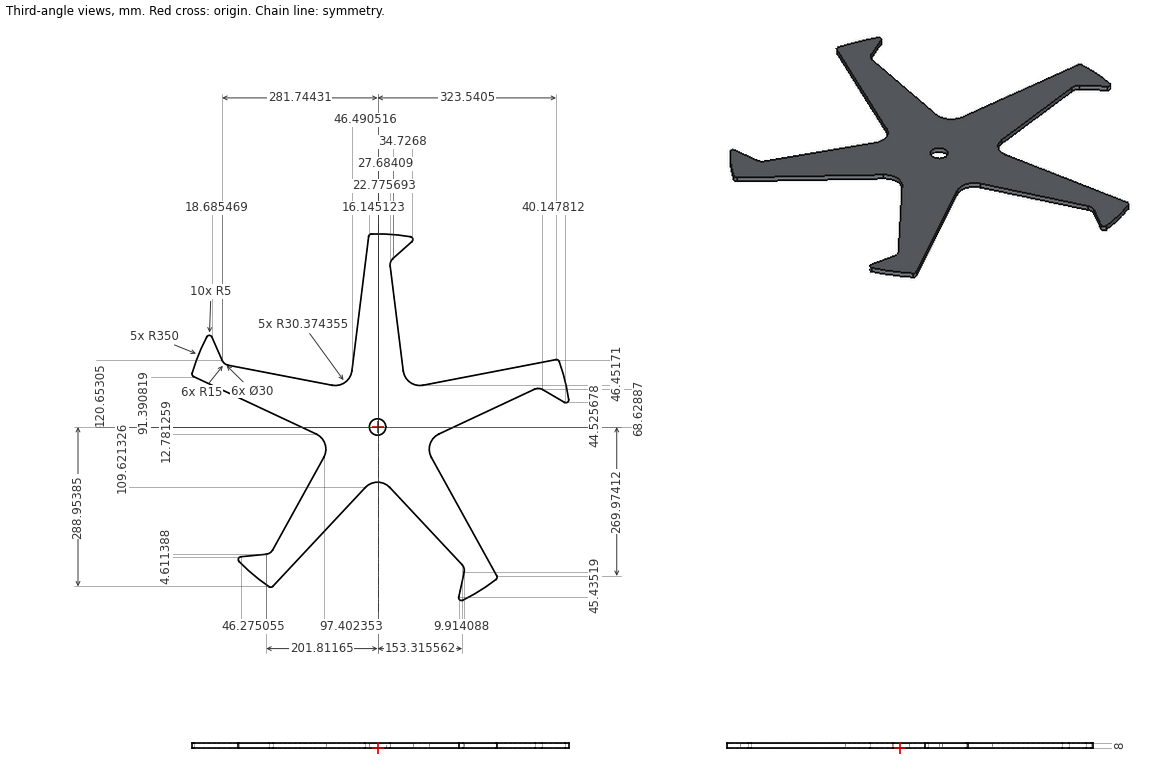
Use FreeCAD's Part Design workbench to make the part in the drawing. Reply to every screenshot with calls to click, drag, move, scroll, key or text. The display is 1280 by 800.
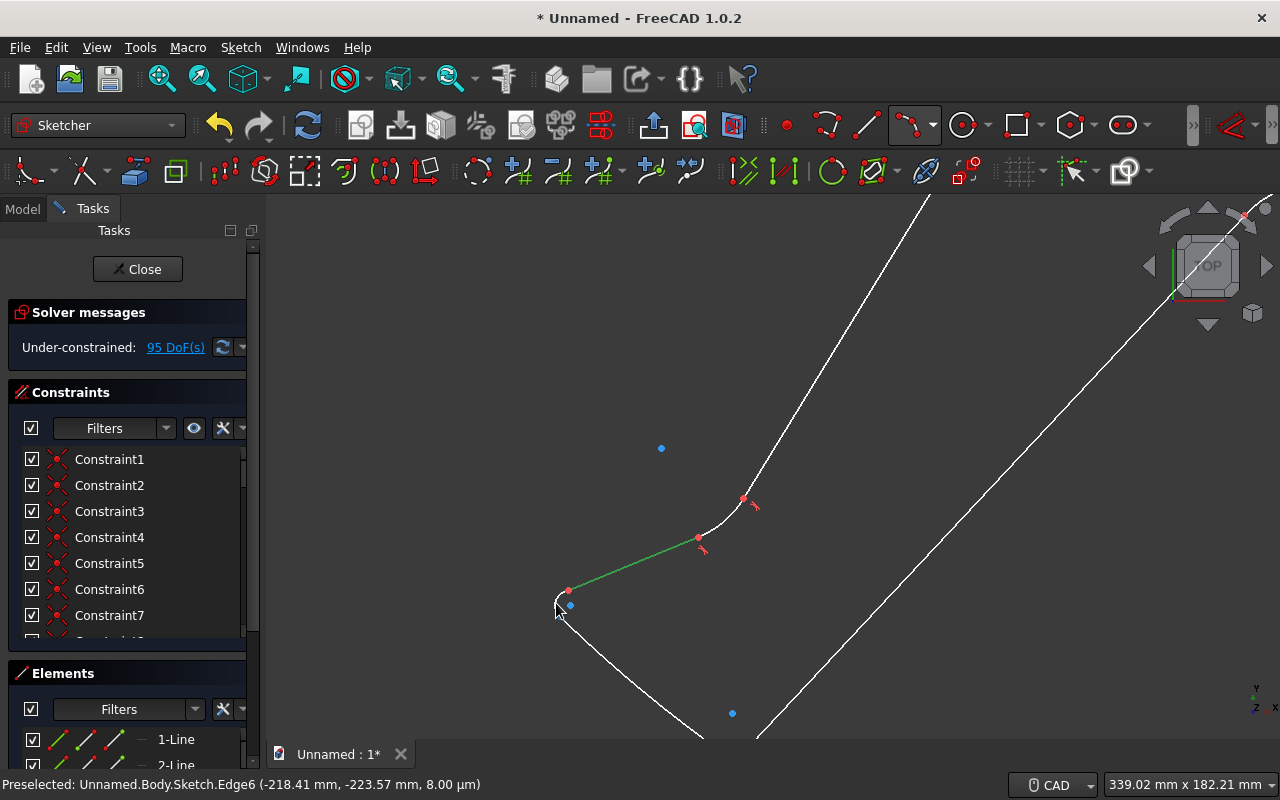
click(556, 601)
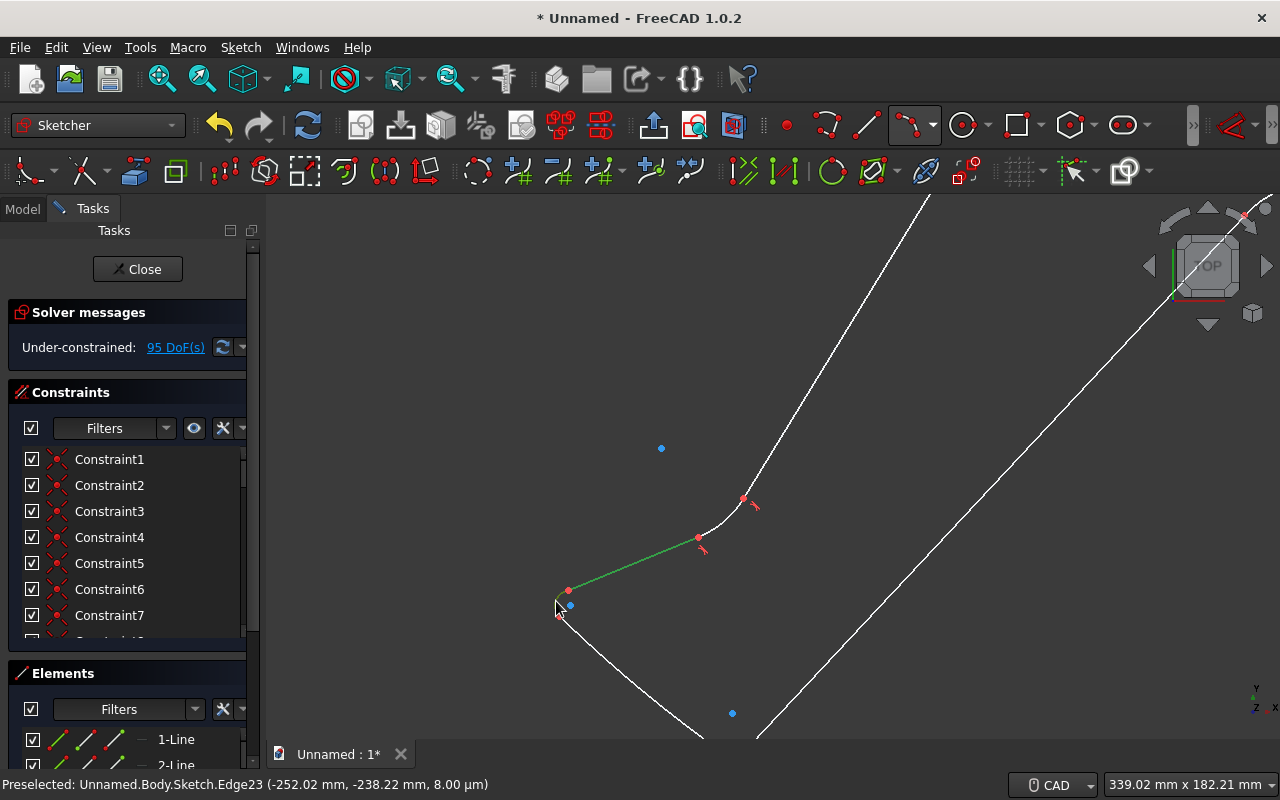
key(t)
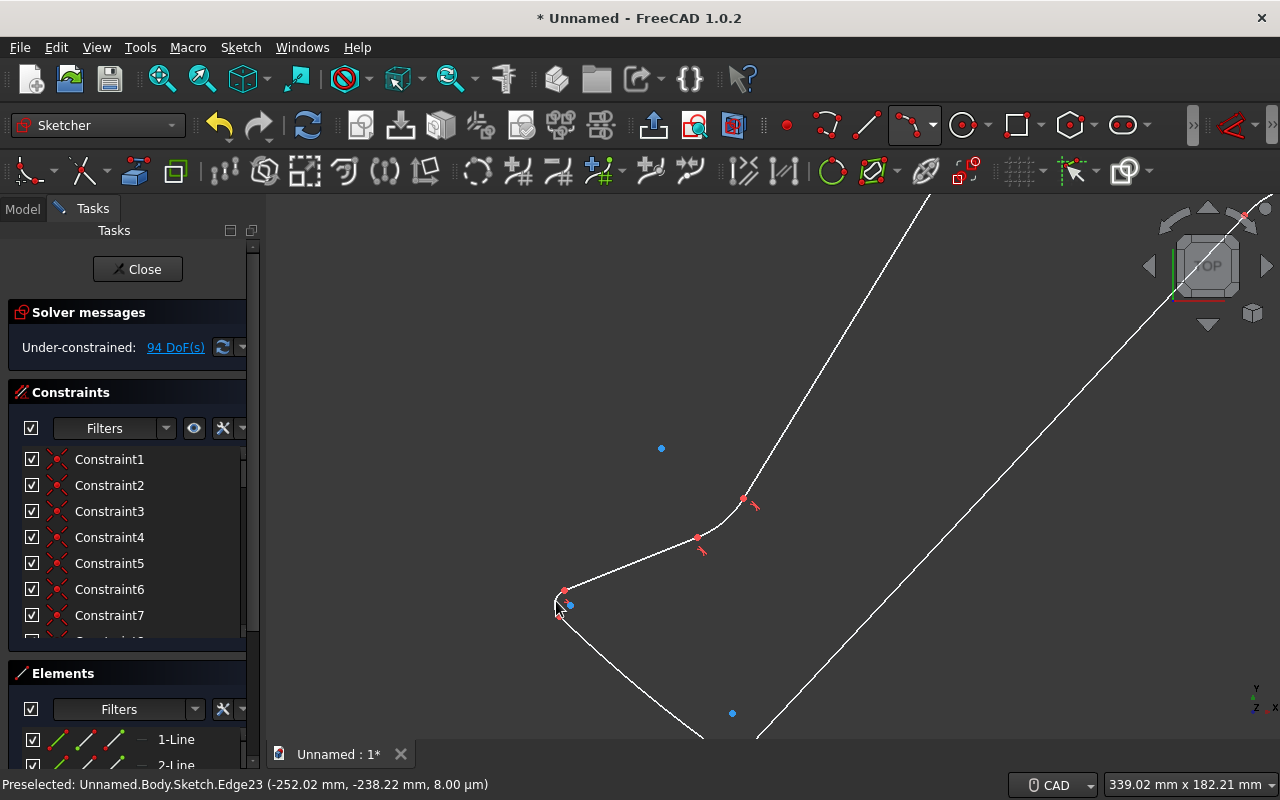
scroll(581, 592, down, 9)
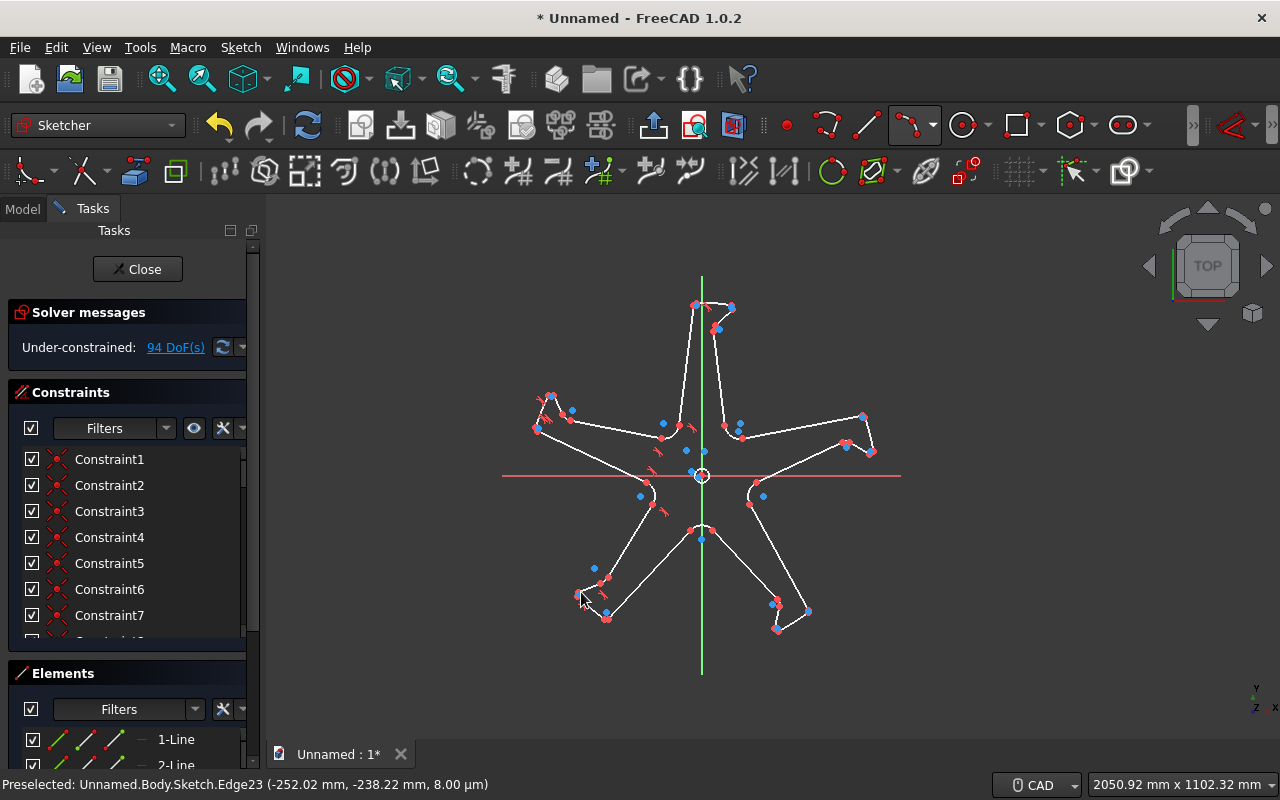
click(633, 593)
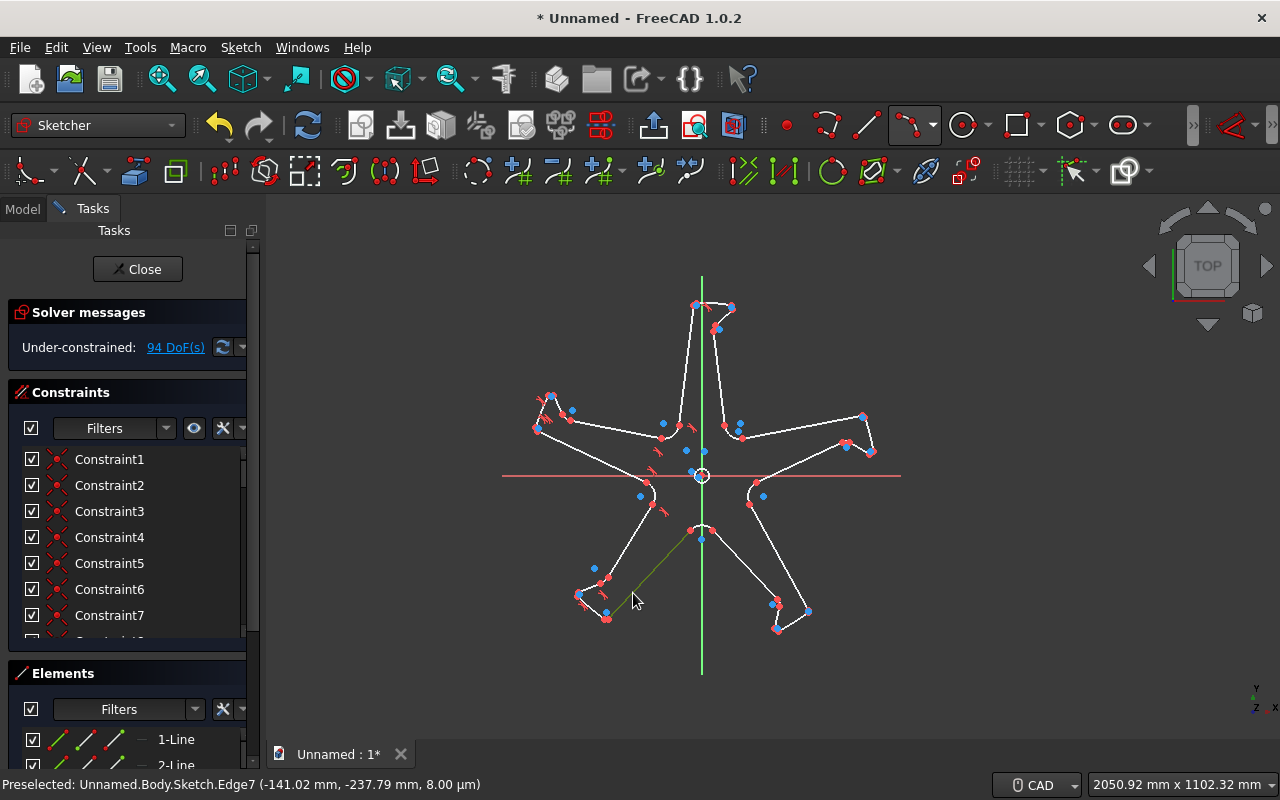
scroll(606, 619, up, 11)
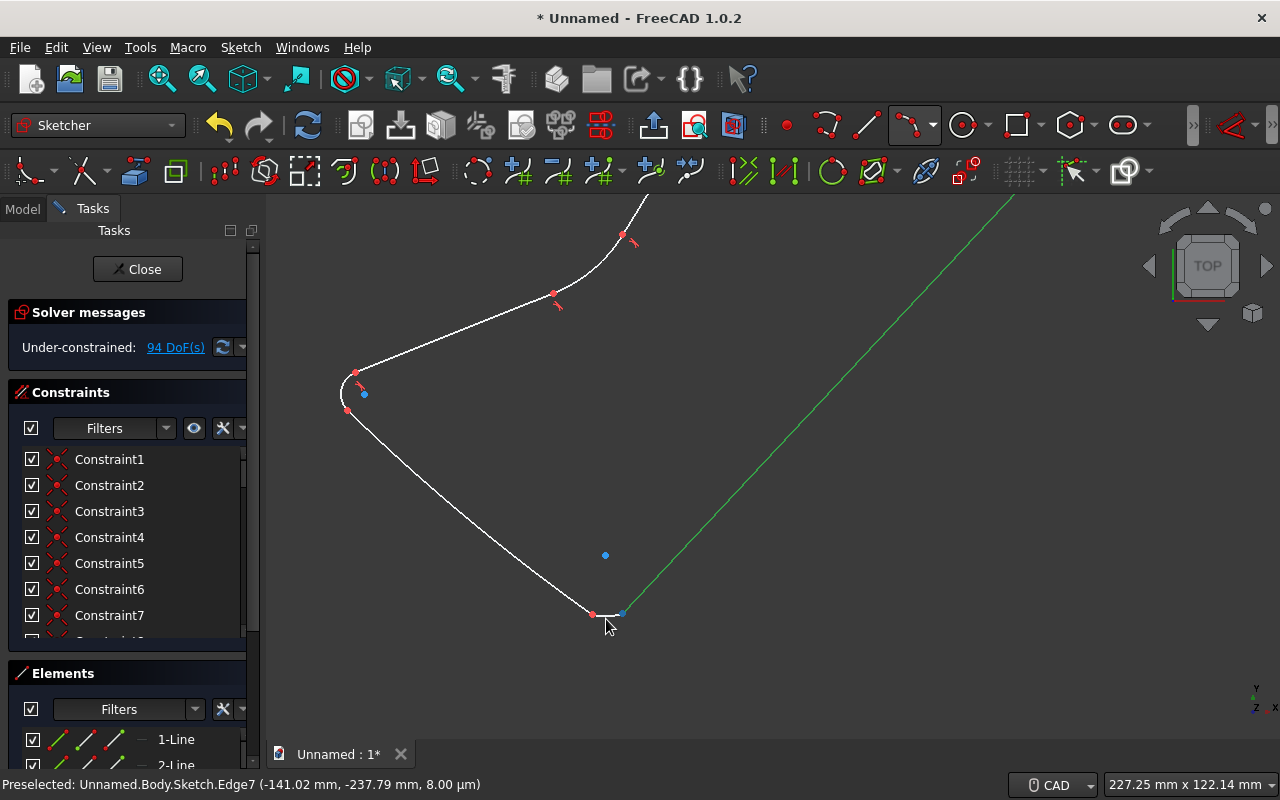
click(607, 616)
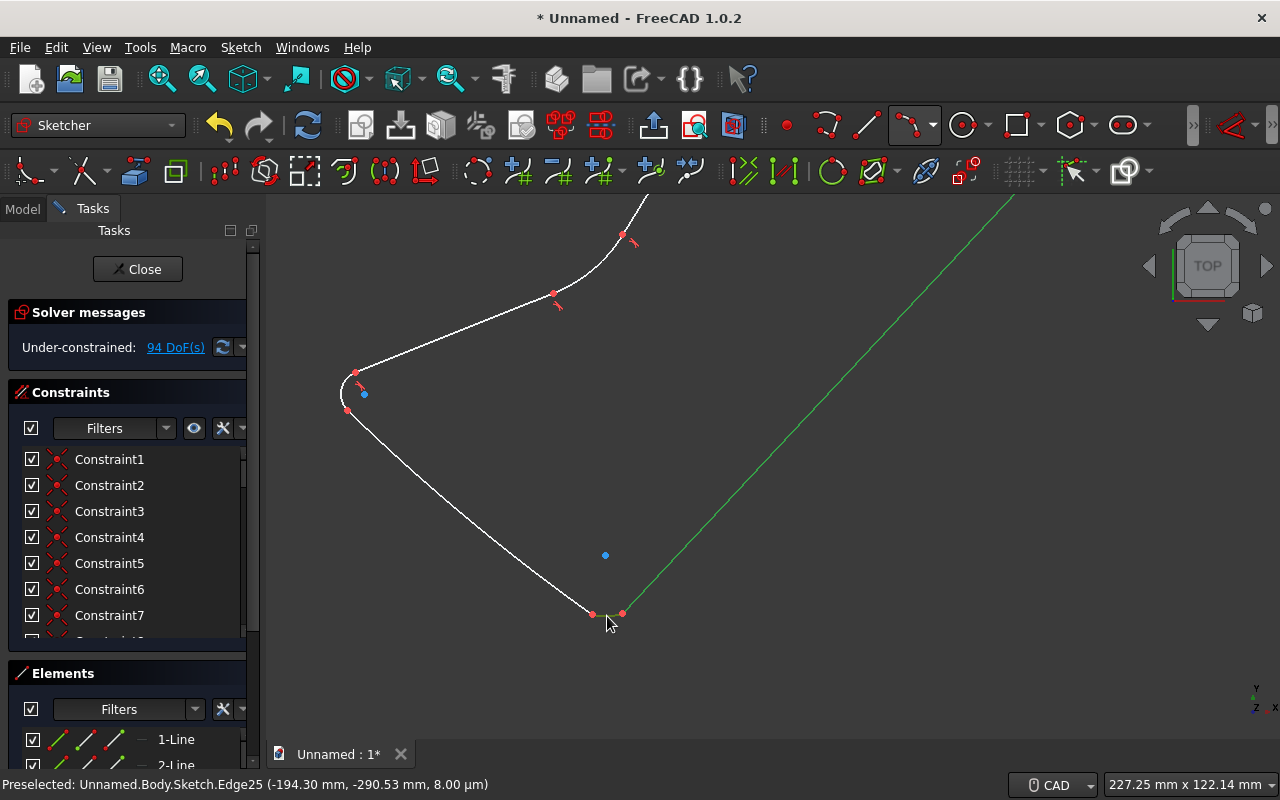
key(t)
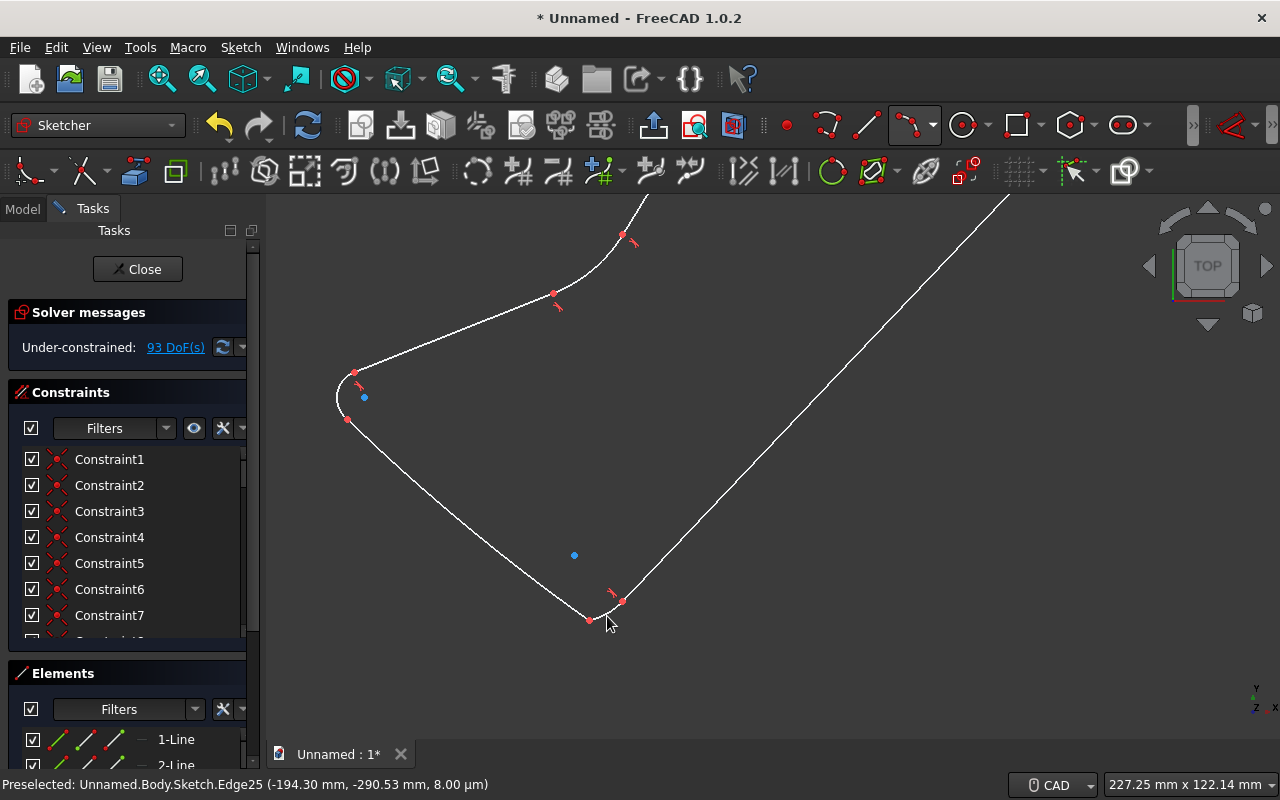
scroll(606, 619, down, 11)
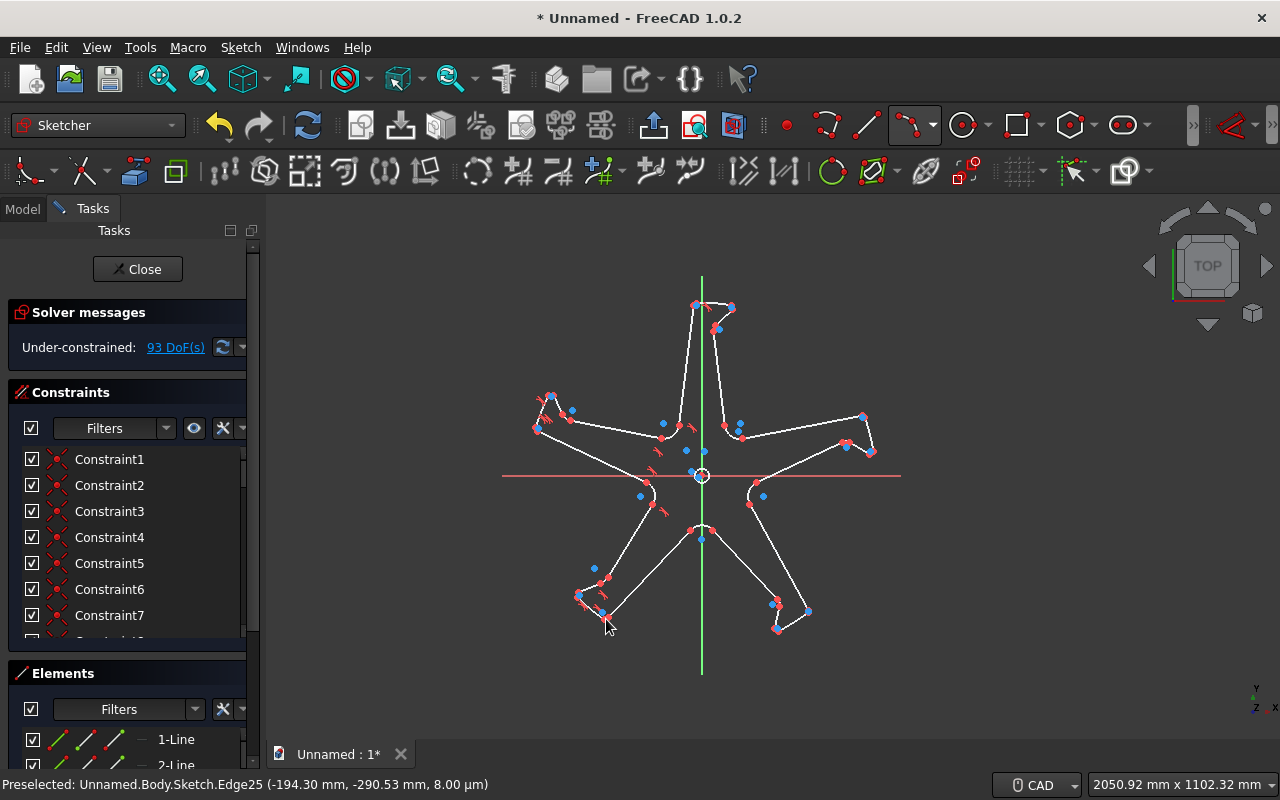
click(633, 592)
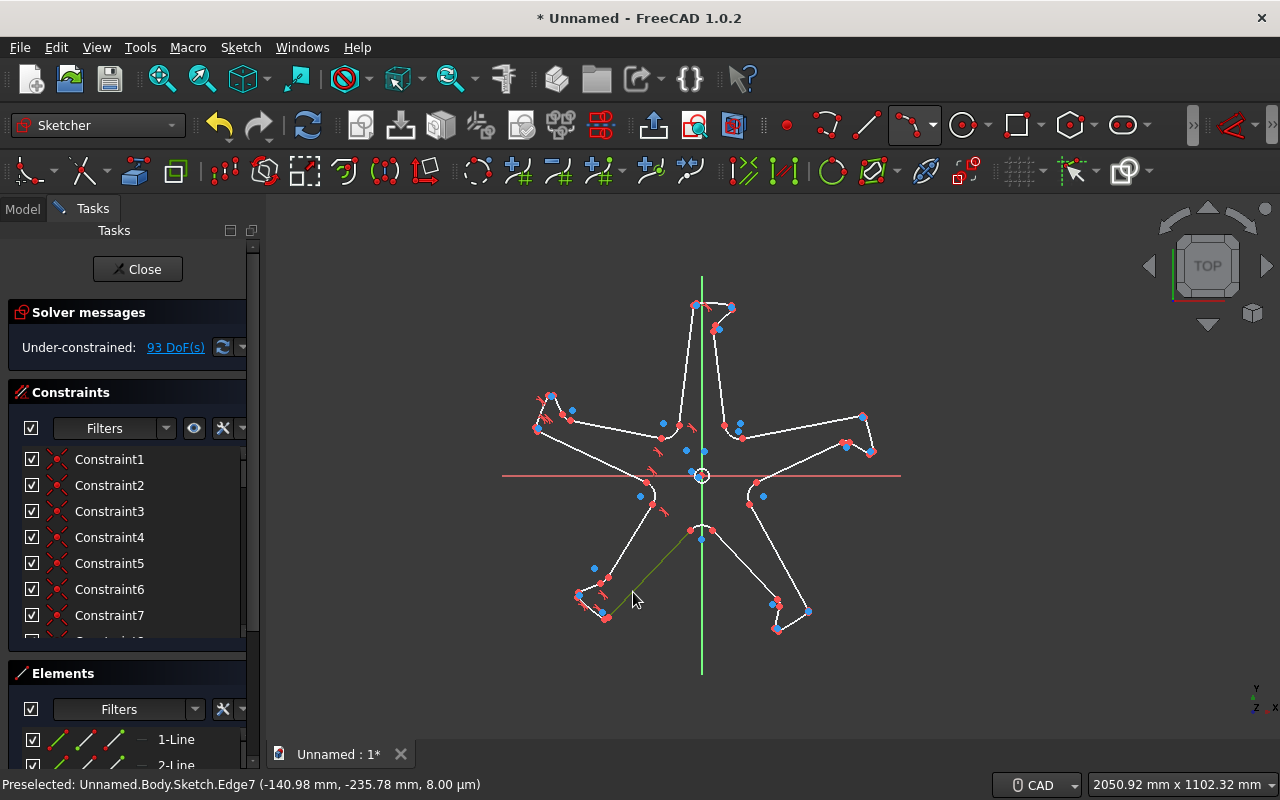
click(702, 525)